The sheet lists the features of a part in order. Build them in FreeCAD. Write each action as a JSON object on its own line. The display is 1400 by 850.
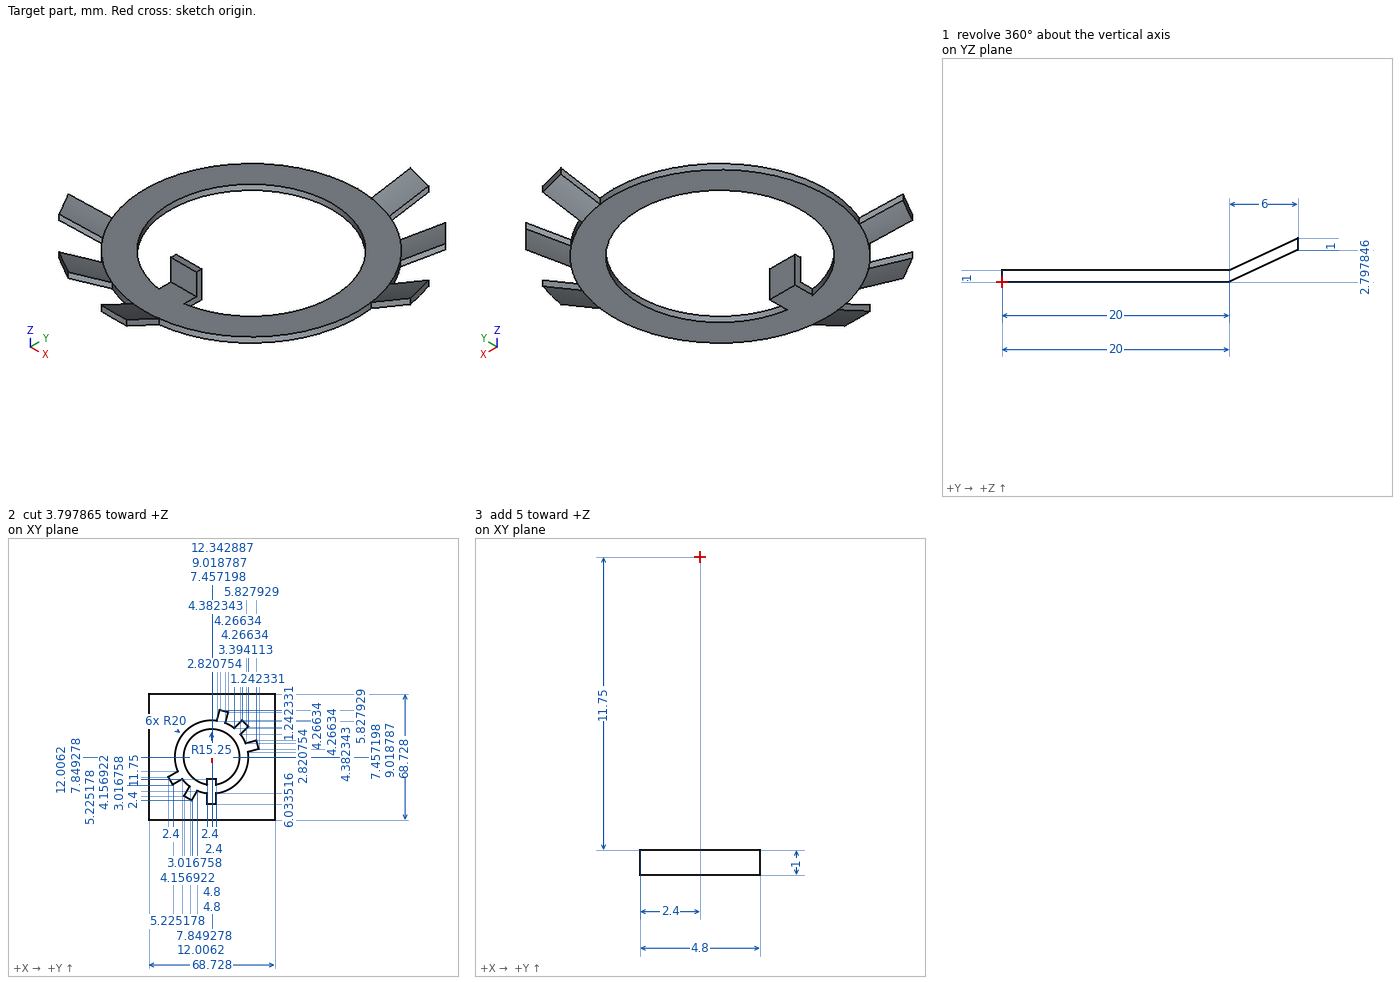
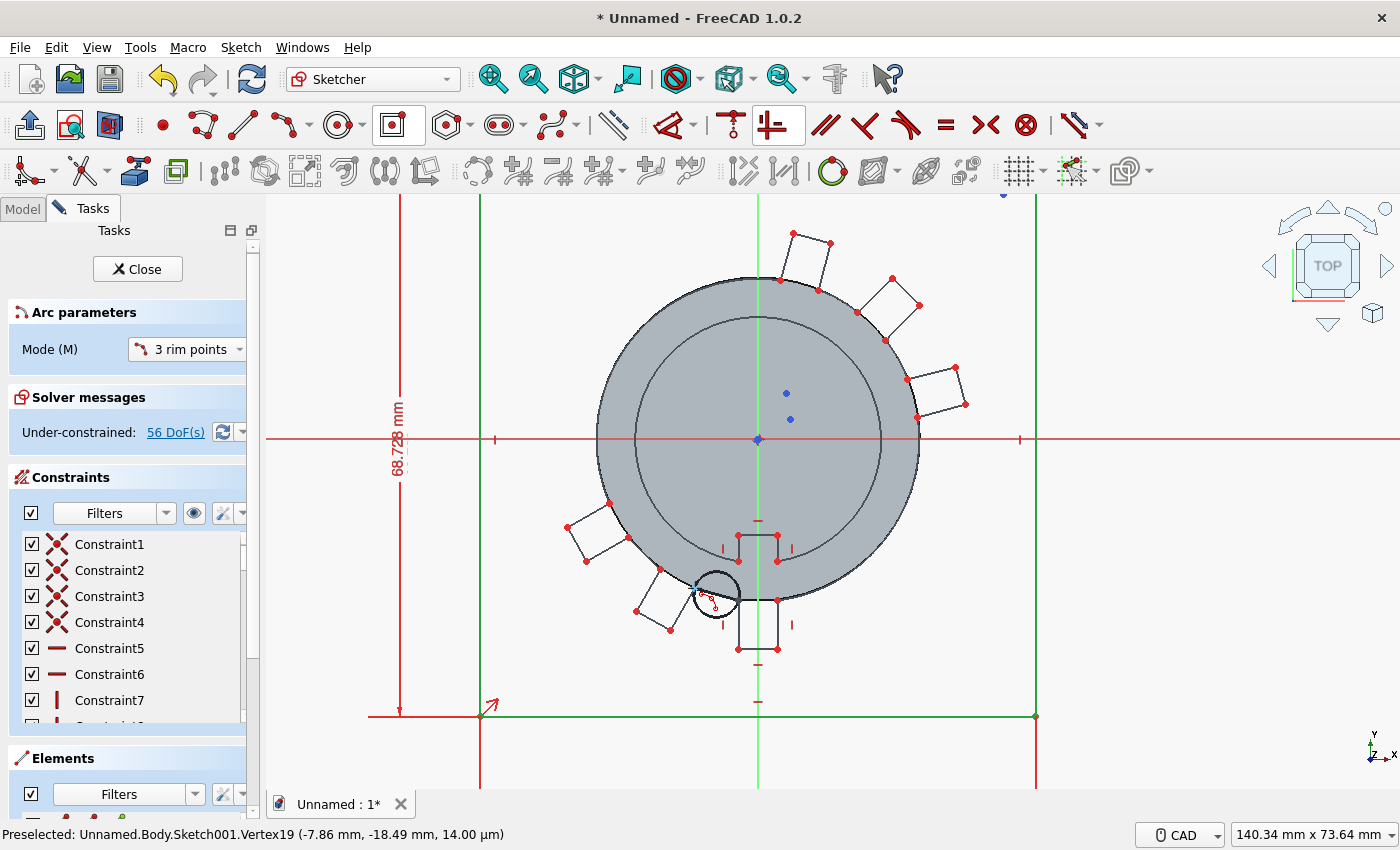
{"action": "scroll", "coordinate": [716, 595], "scroll_direction": "up", "scroll_amount": 12}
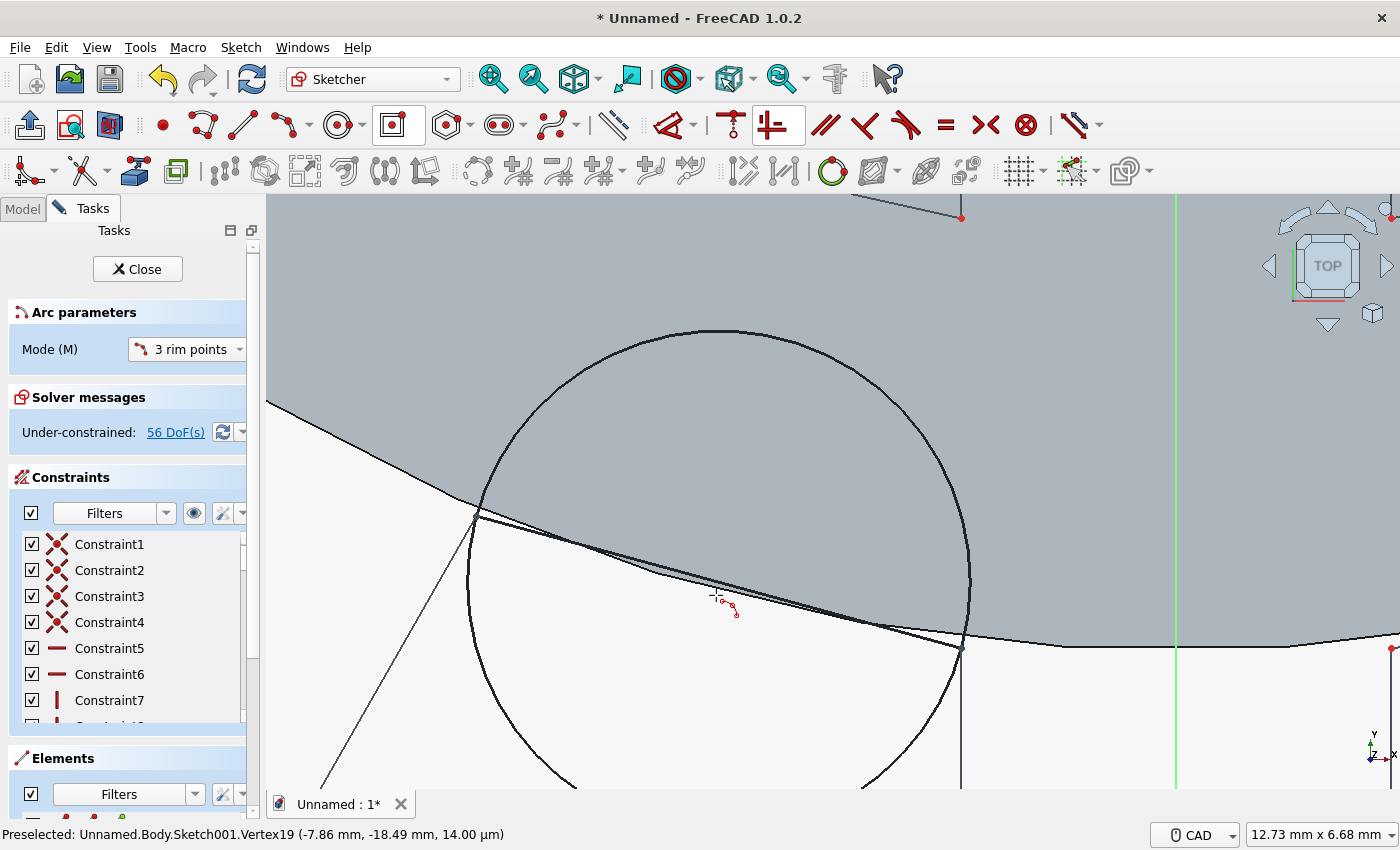
{"action": "left_click", "coordinate": [715, 590]}
{"action": "key", "text": "Escape"}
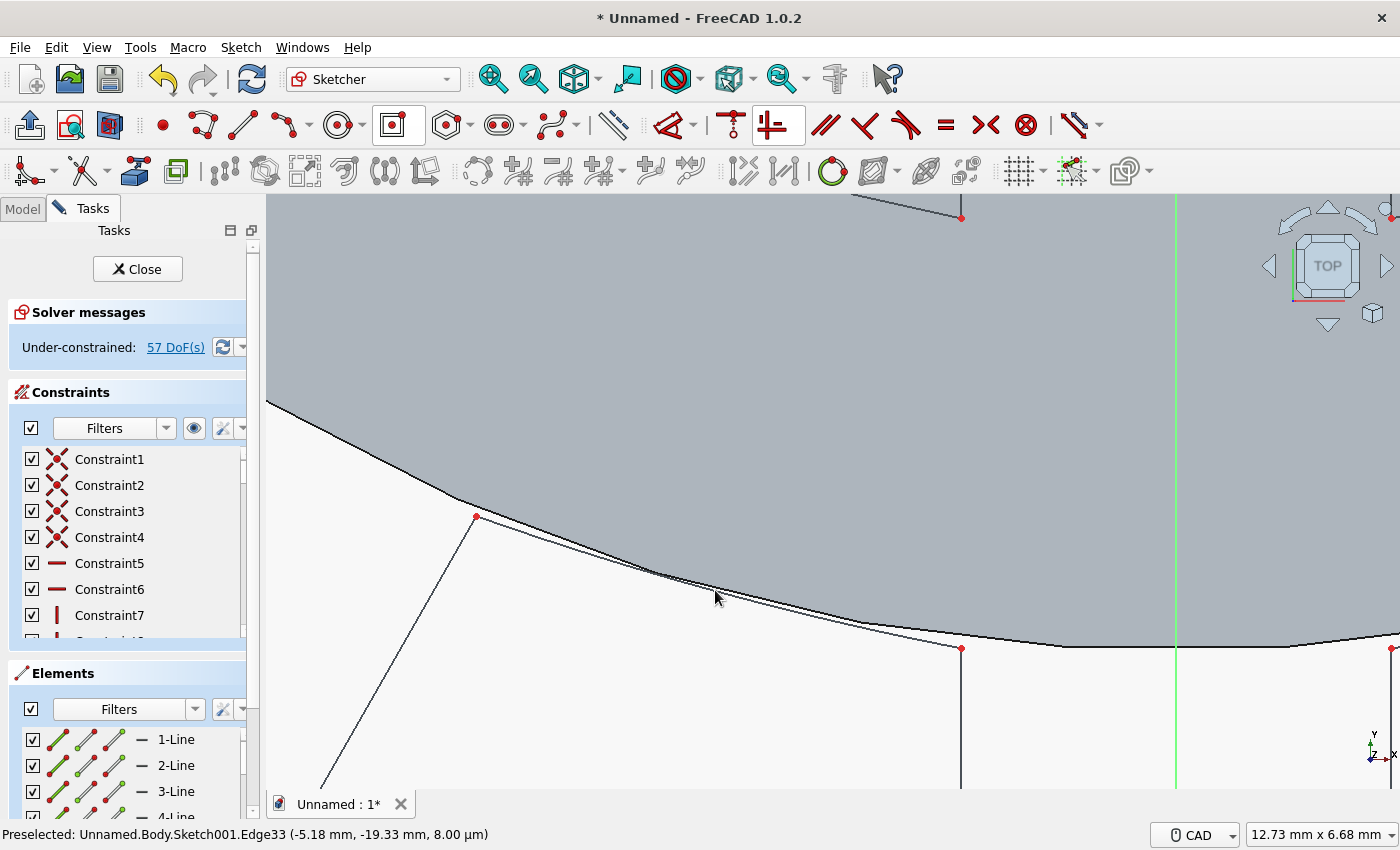
{"action": "scroll", "coordinate": [738, 597], "scroll_direction": "down", "scroll_amount": 14}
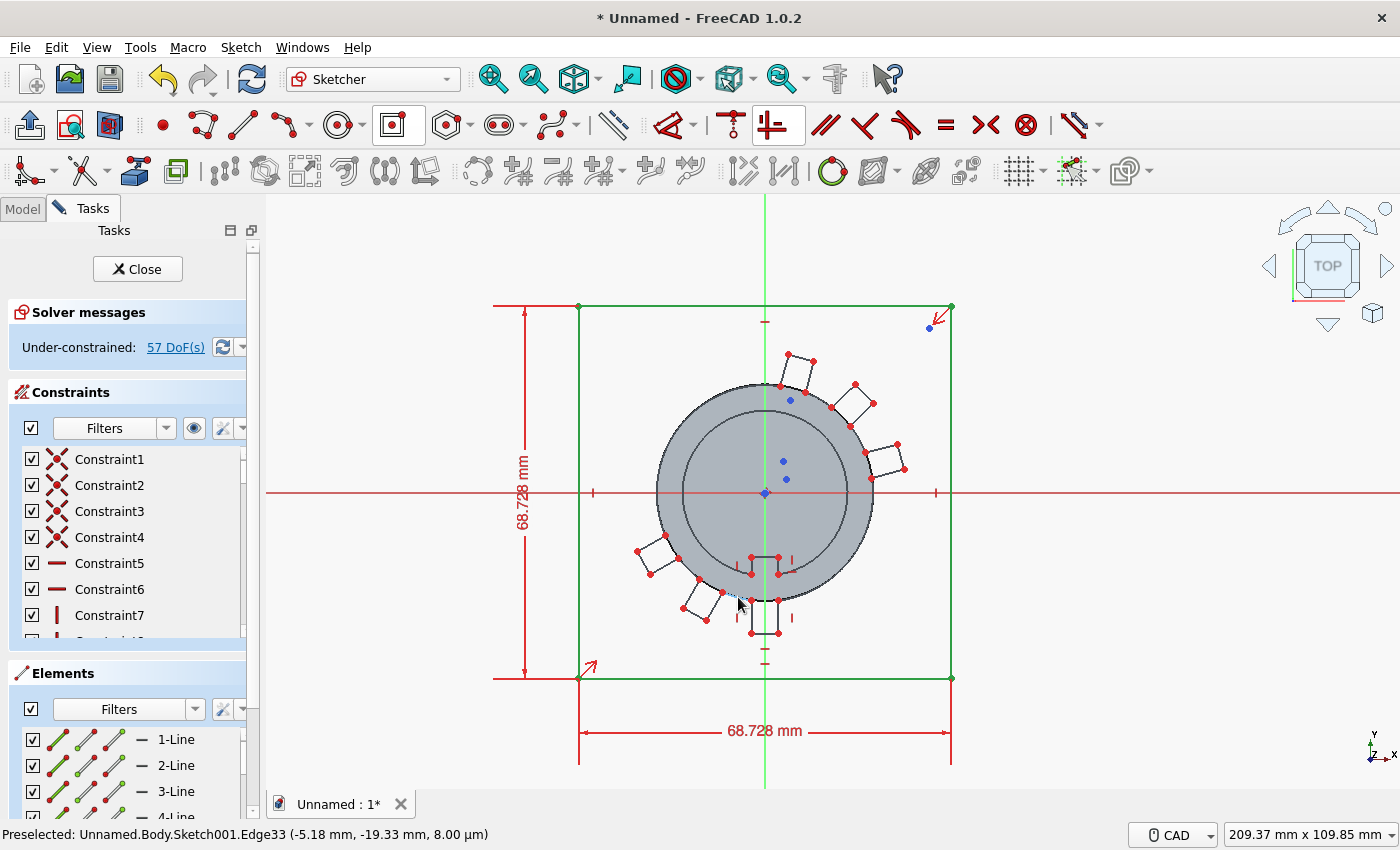
{"action": "left_click", "coordinate": [842, 463]}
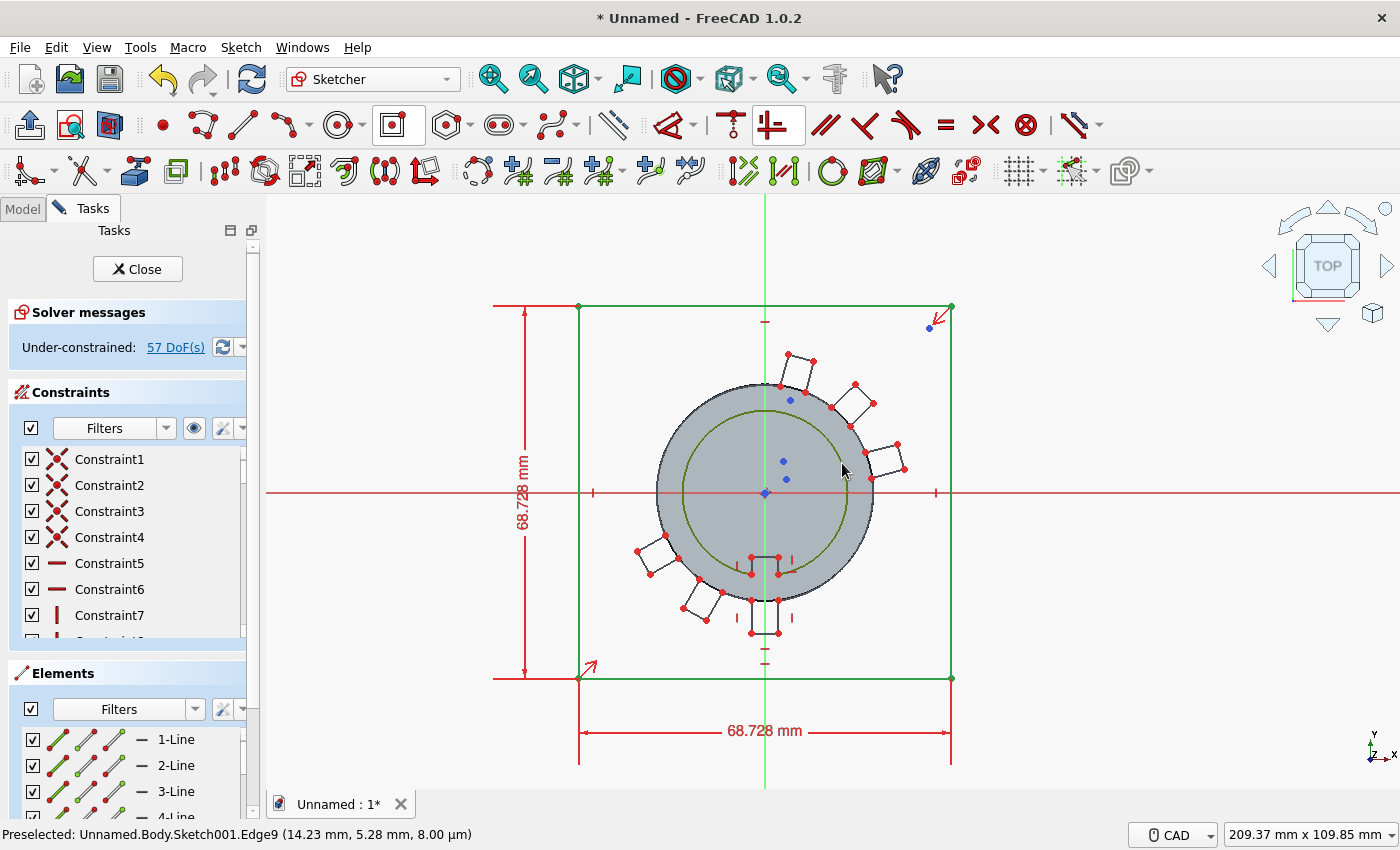
{"action": "scroll", "coordinate": [684, 565], "scroll_direction": "up", "scroll_amount": 3}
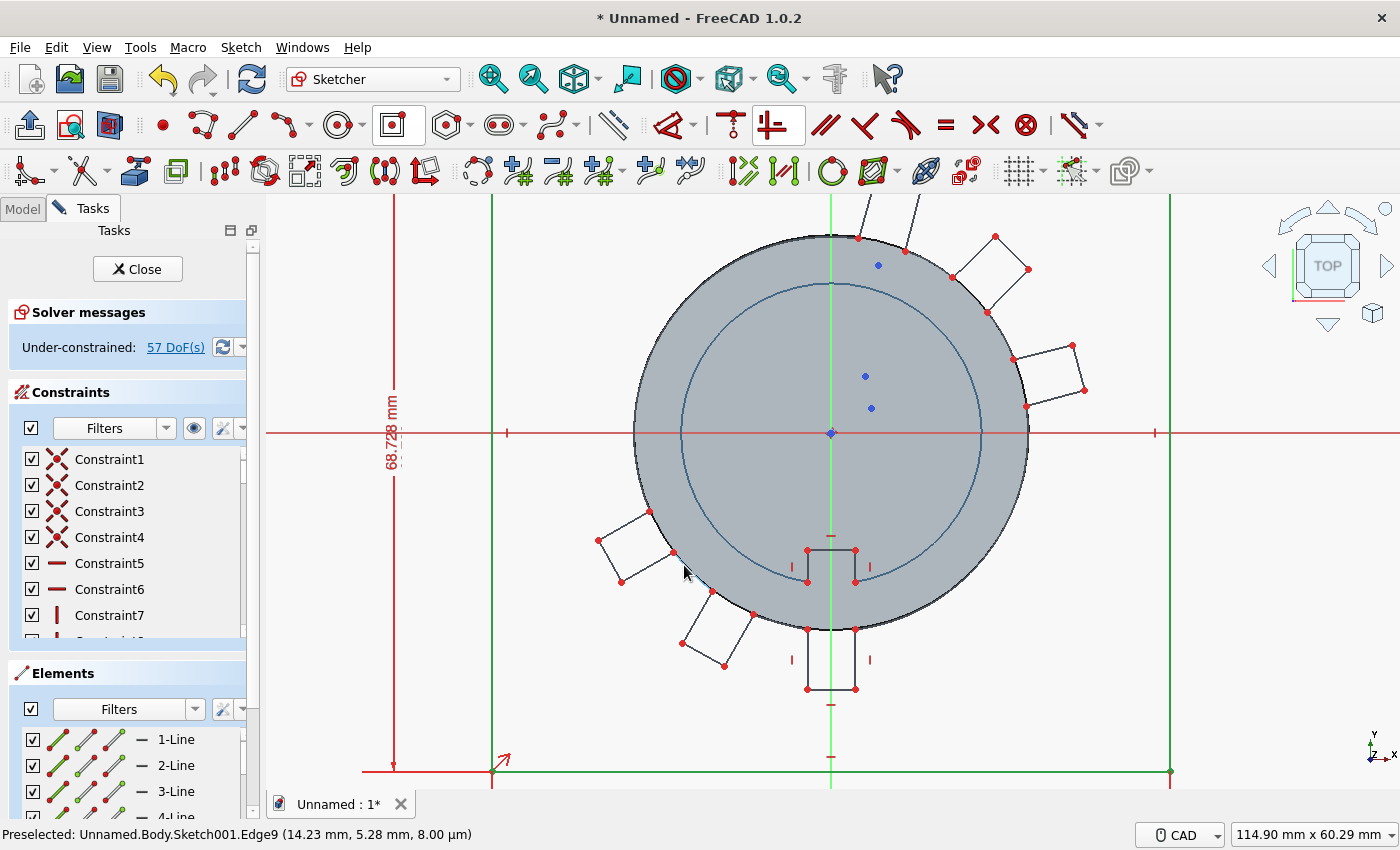
{"action": "left_click", "coordinate": [685, 565]}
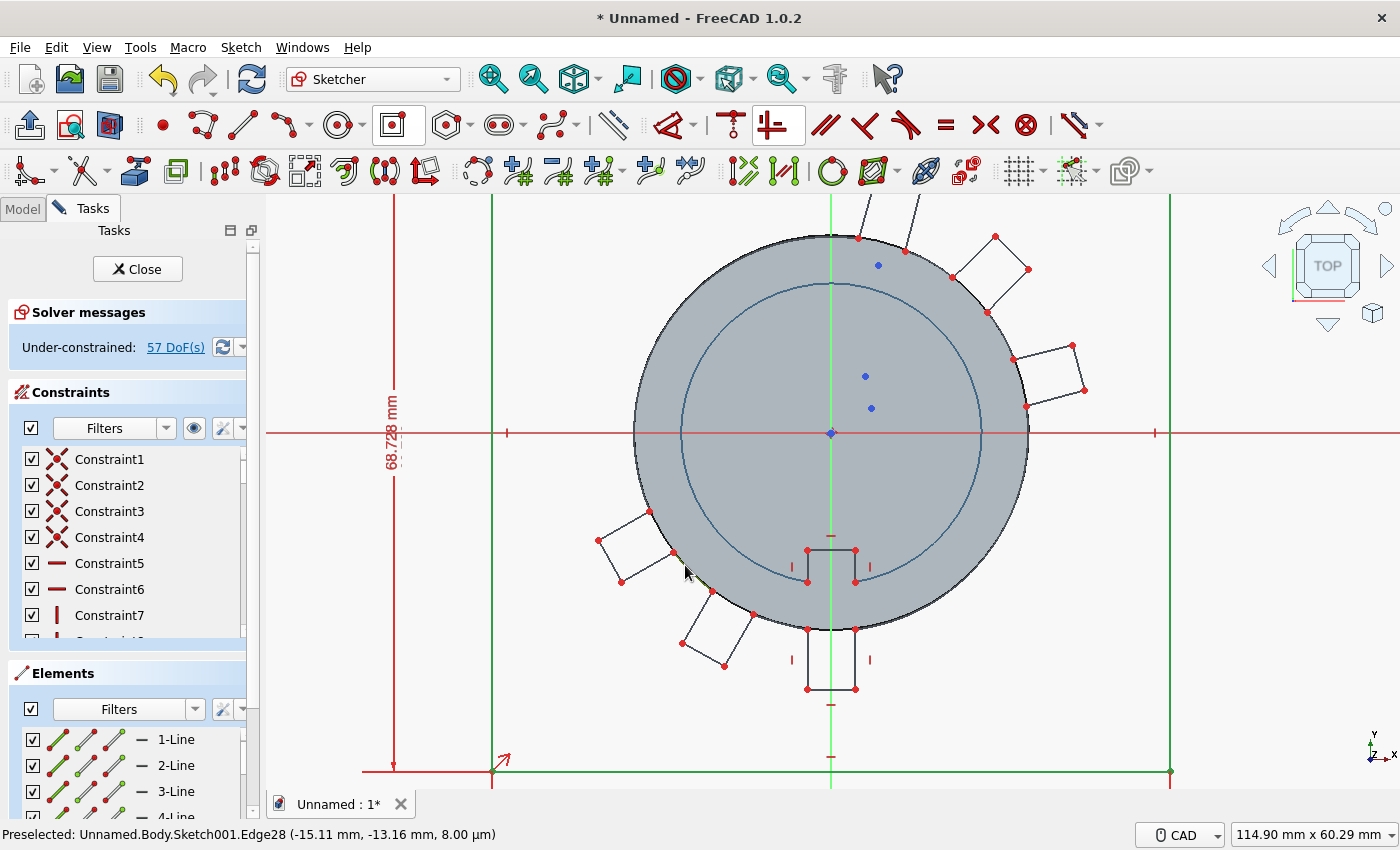
{"action": "left_click", "coordinate": [732, 126]}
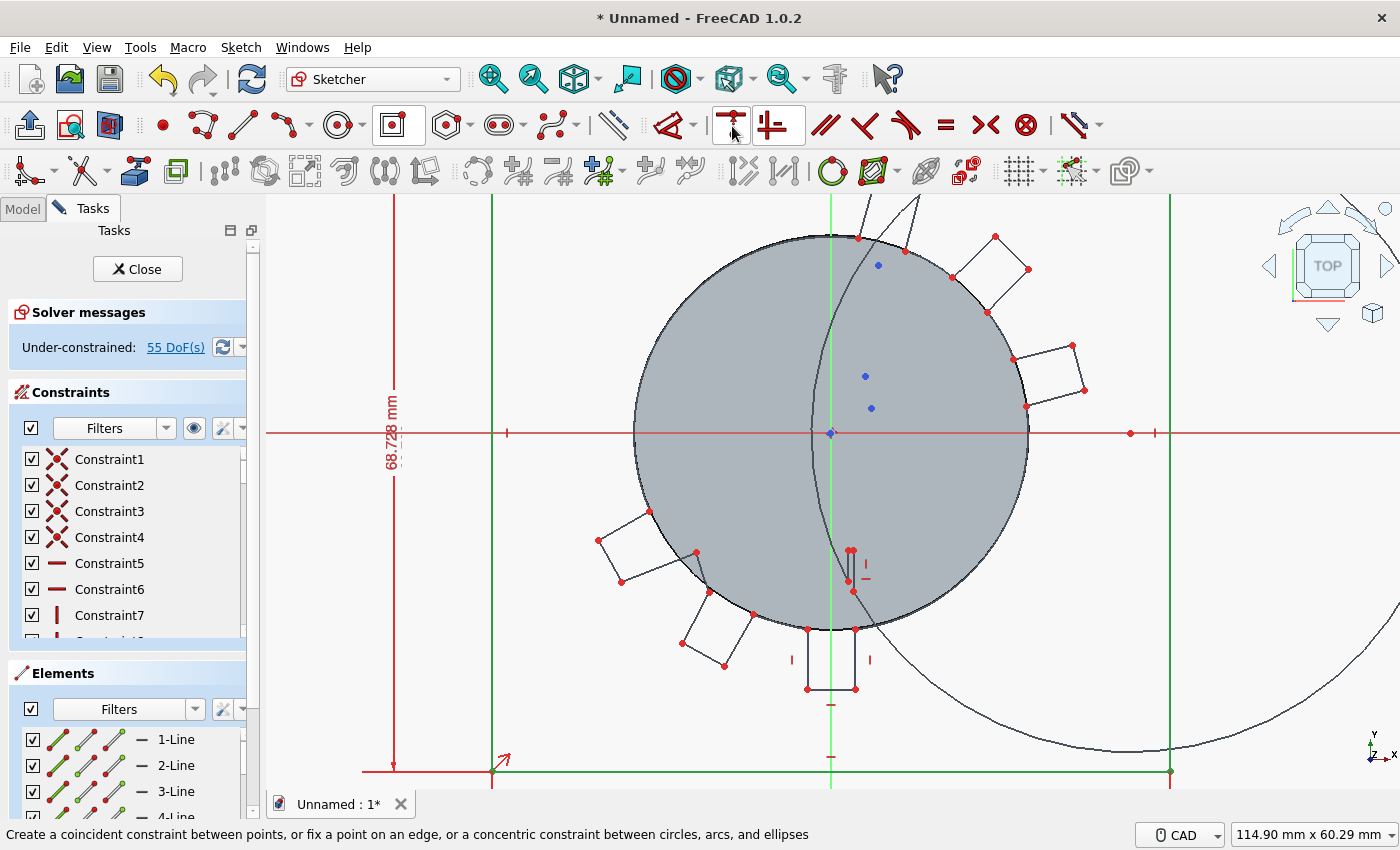
{"action": "left_click", "coordinate": [1193, 746]}